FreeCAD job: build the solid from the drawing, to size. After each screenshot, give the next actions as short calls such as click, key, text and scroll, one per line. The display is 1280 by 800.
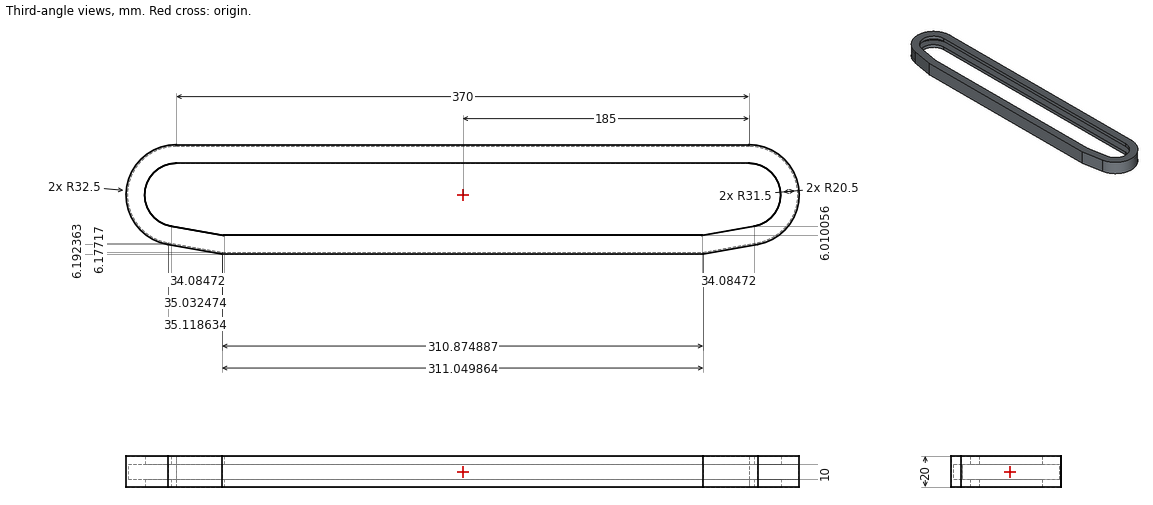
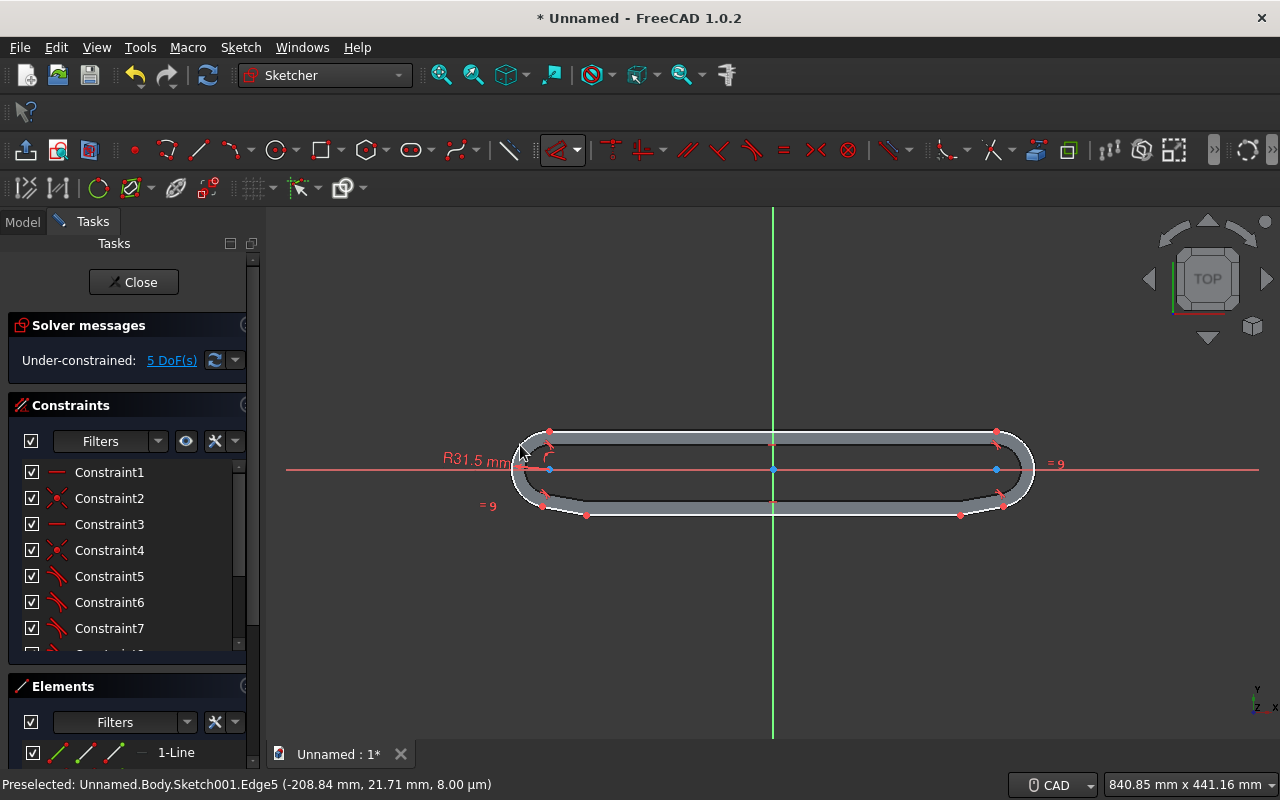
click(862, 432)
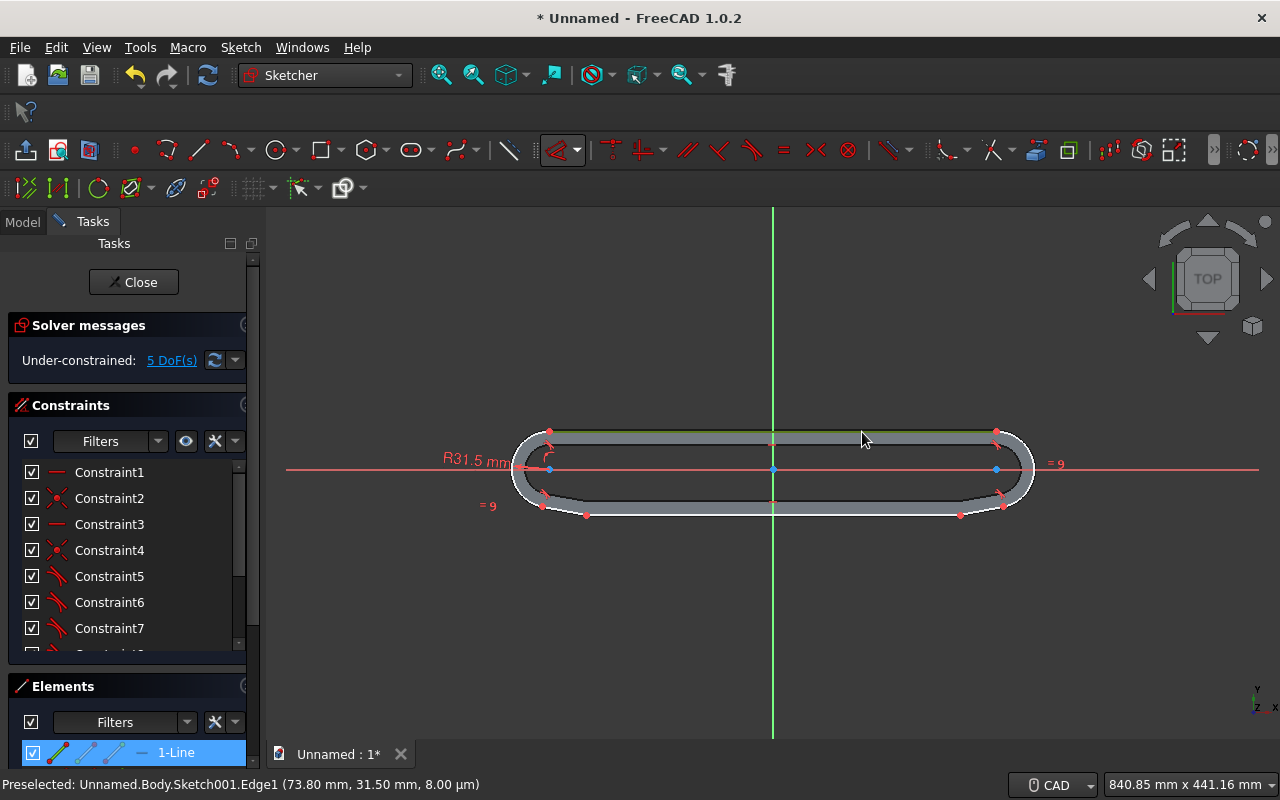
click(580, 150)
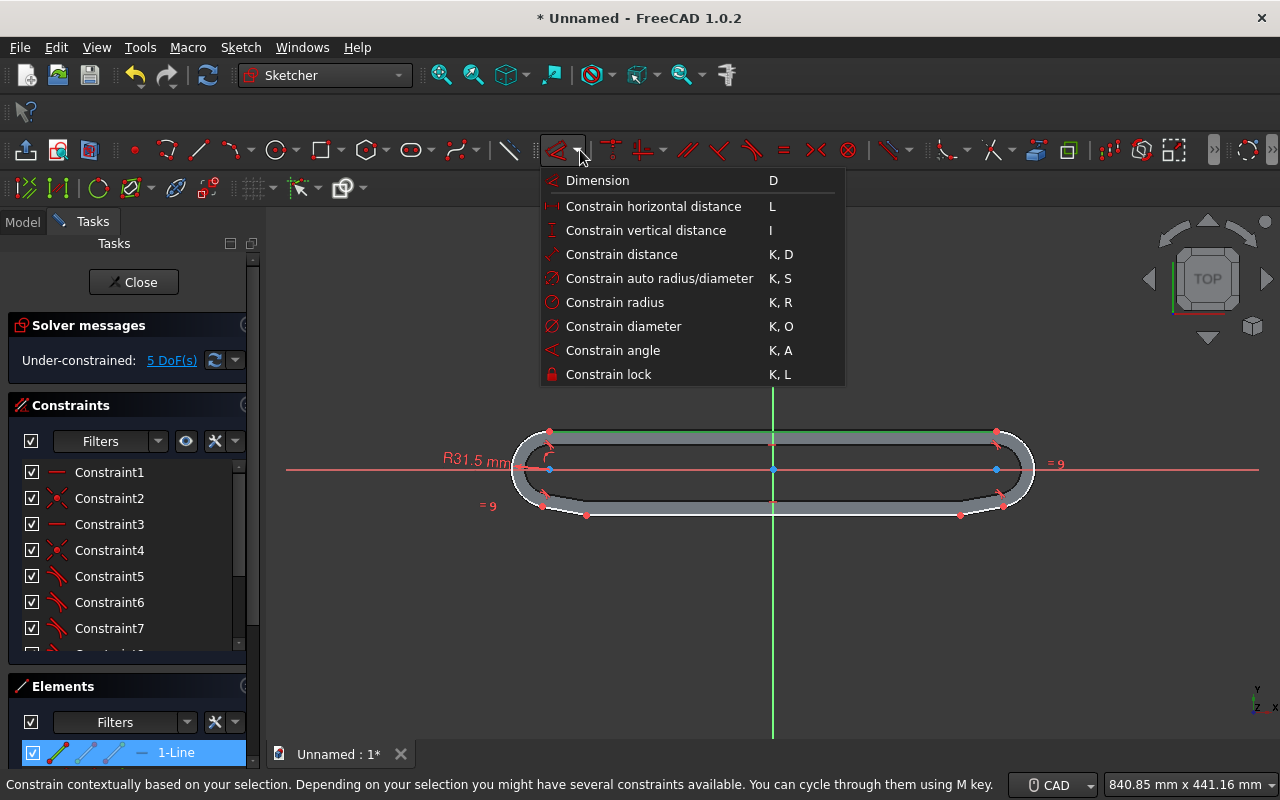
click(693, 206)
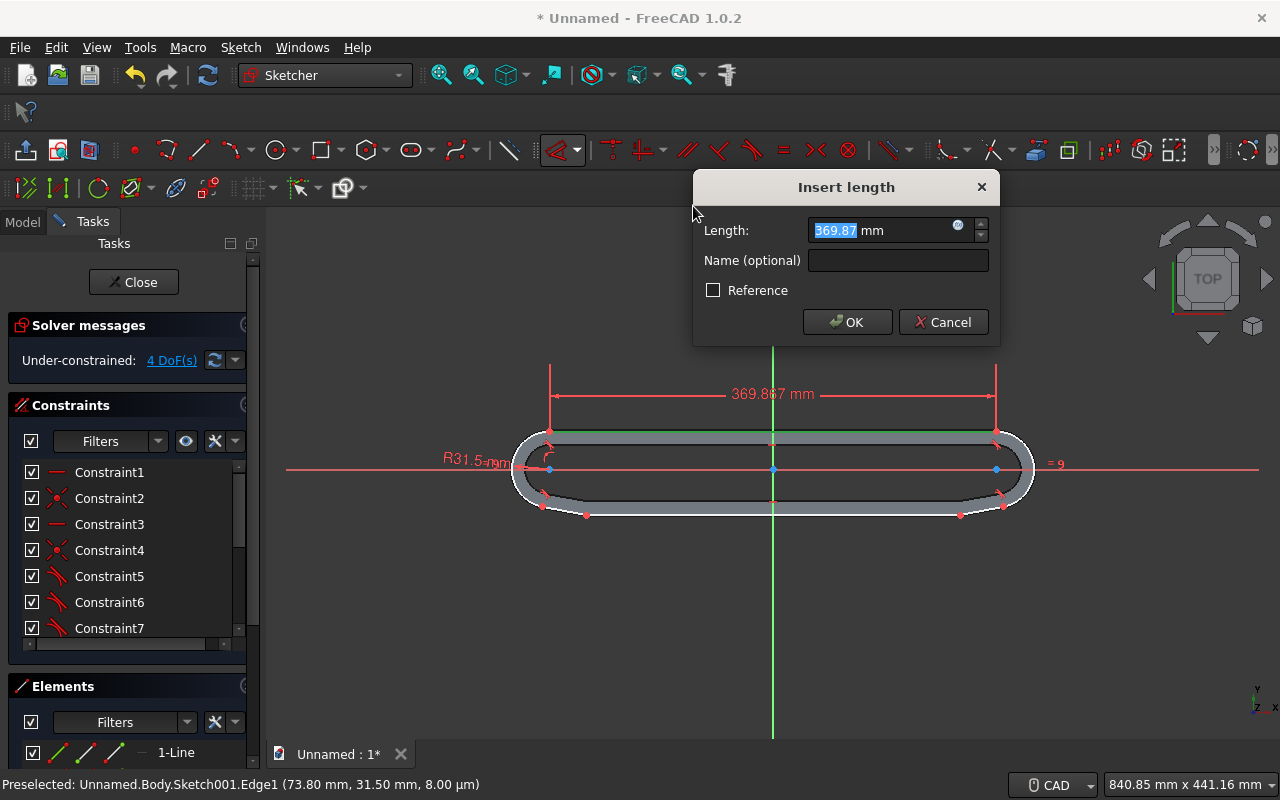
text(370)
key(Return)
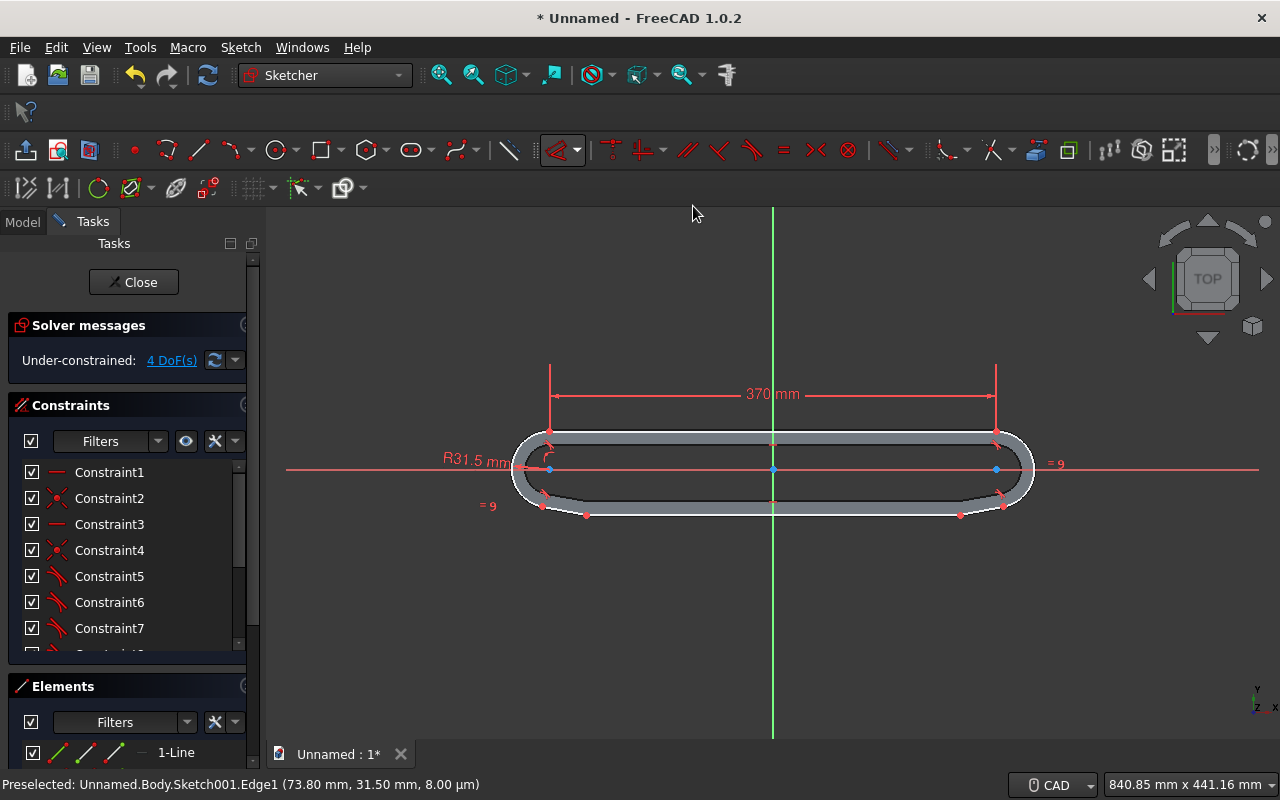
click(996, 432)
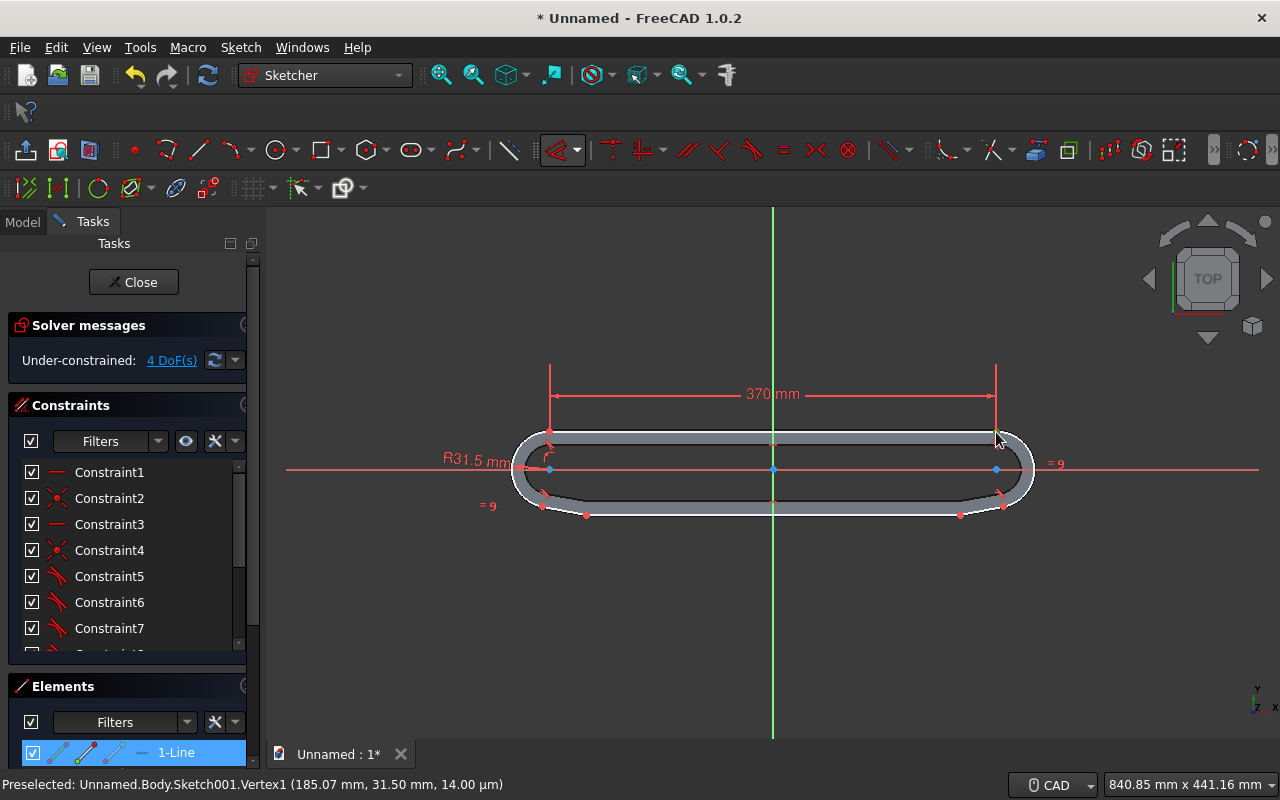
key(l)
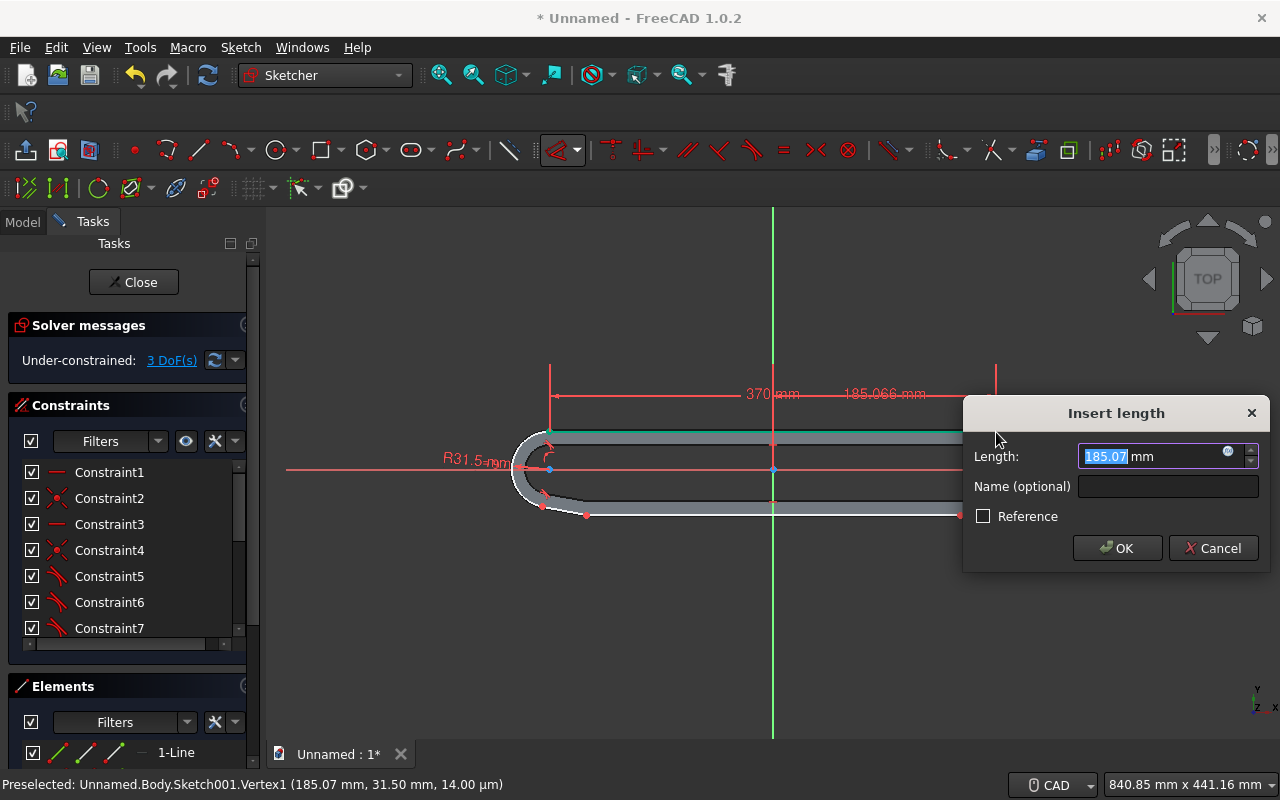
text(185)
key(Return)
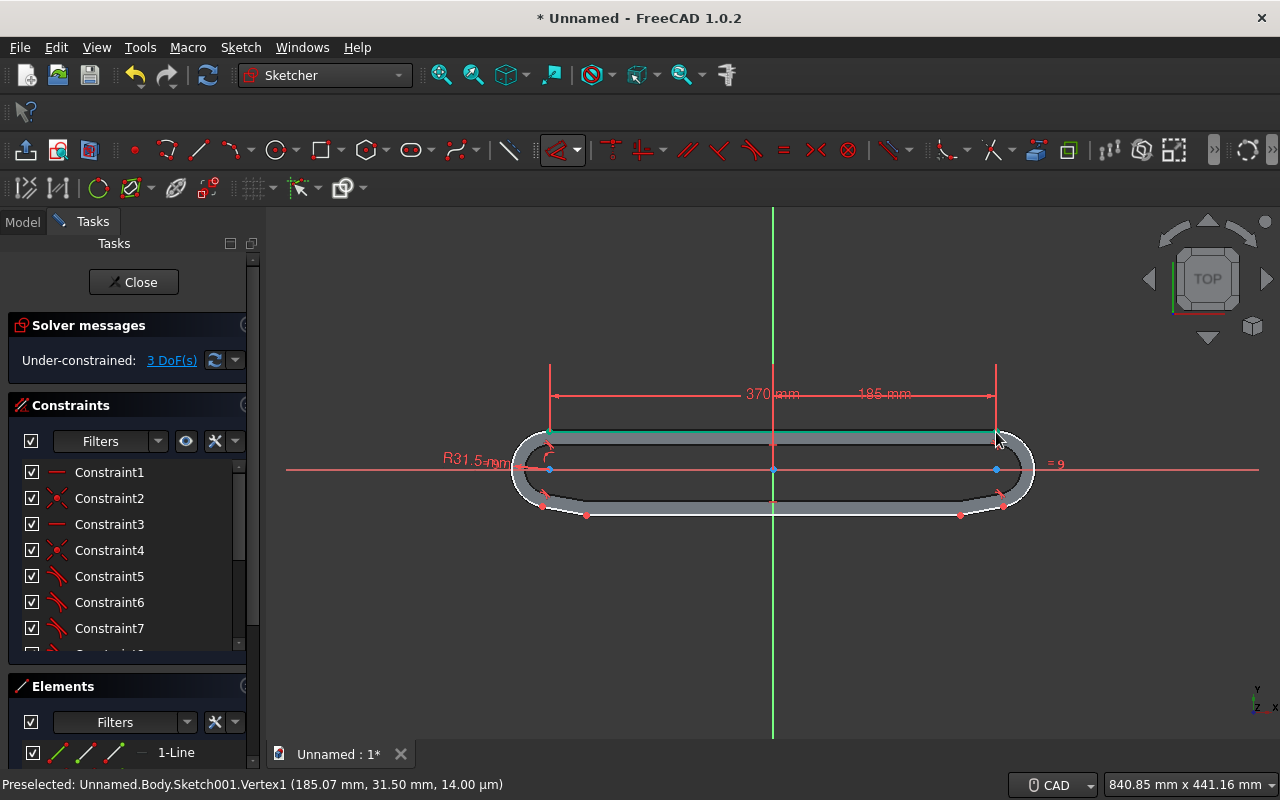
scroll(556, 509, up, 9)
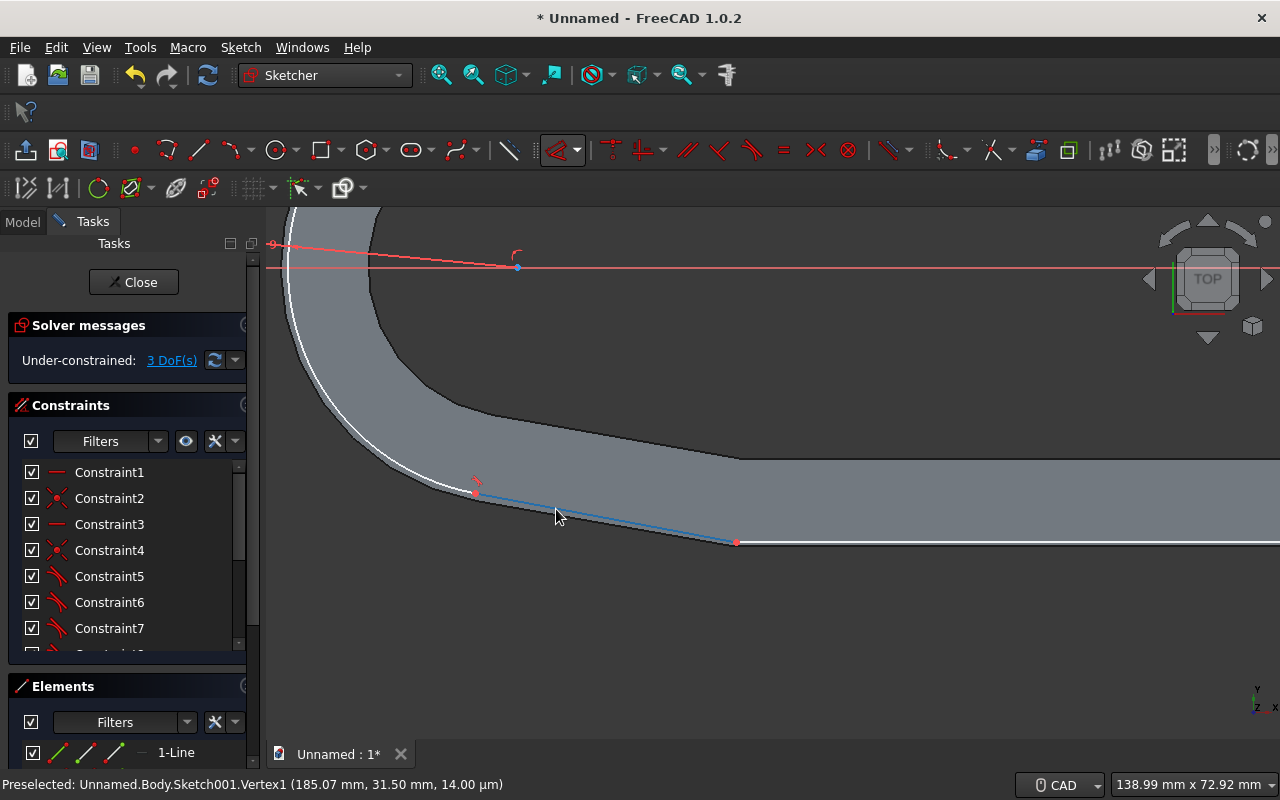
click(553, 508)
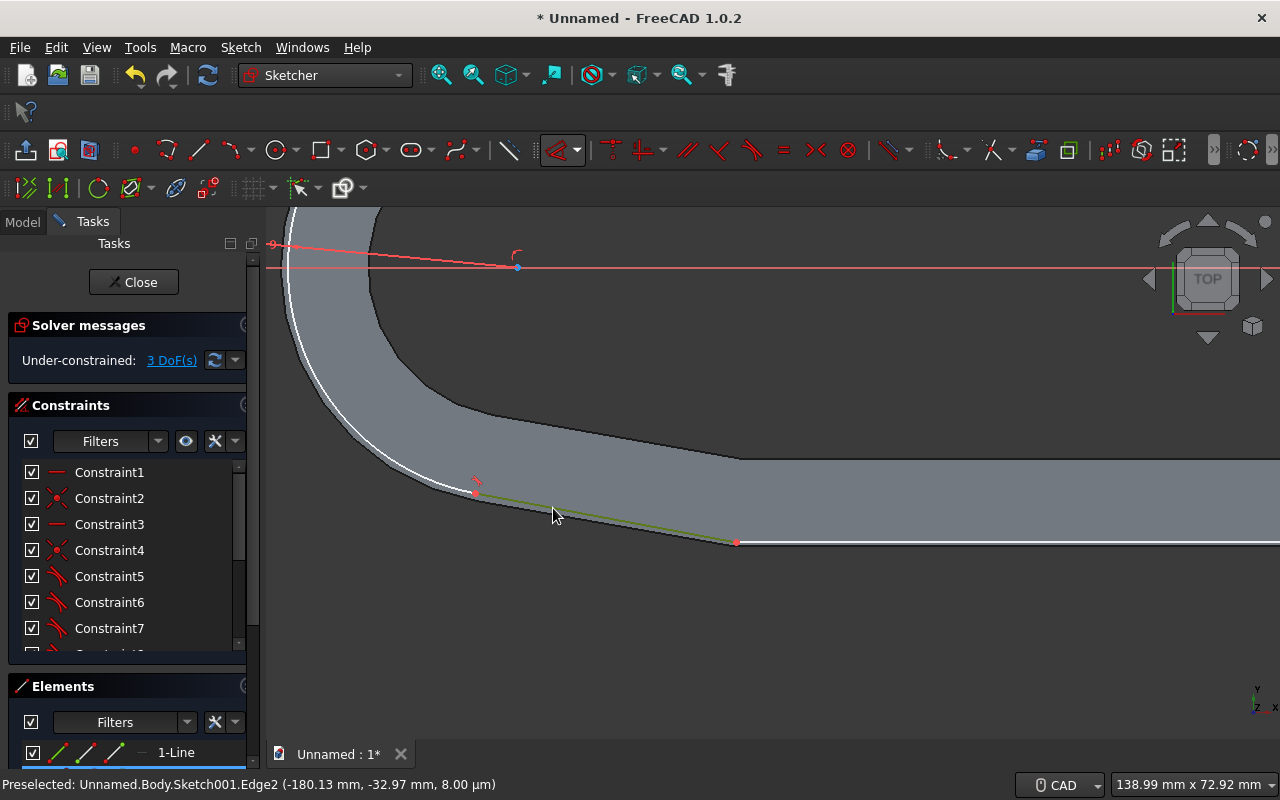
key(i)